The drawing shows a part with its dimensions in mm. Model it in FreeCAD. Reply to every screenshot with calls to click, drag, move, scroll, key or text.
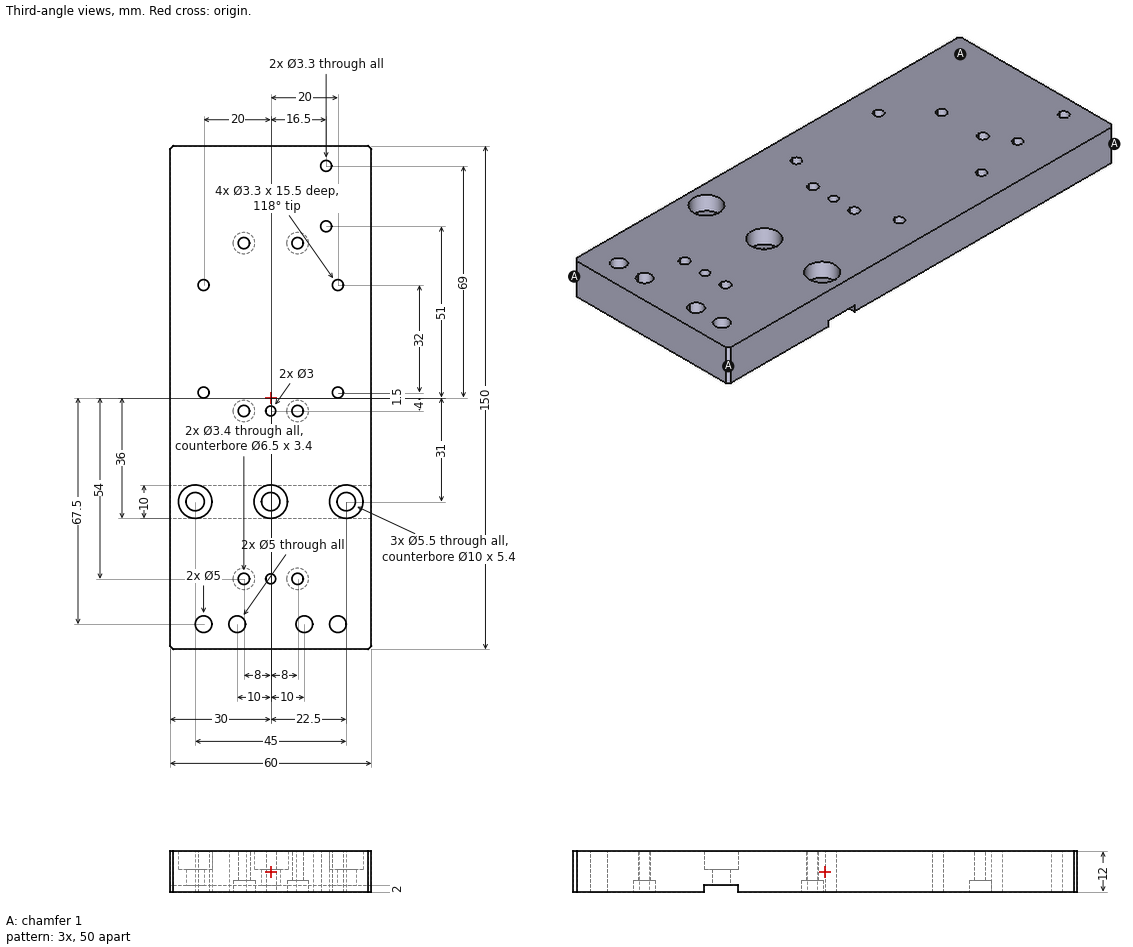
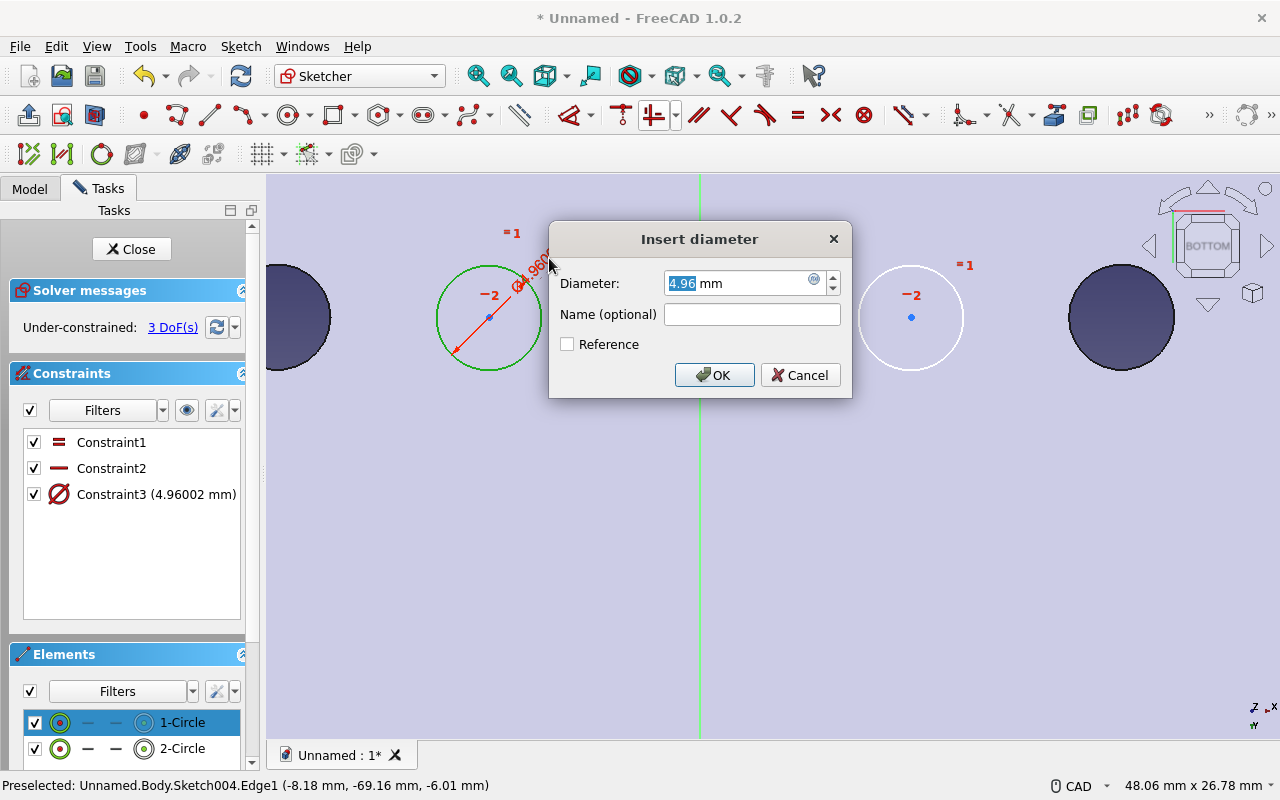
text(5)
key(Return)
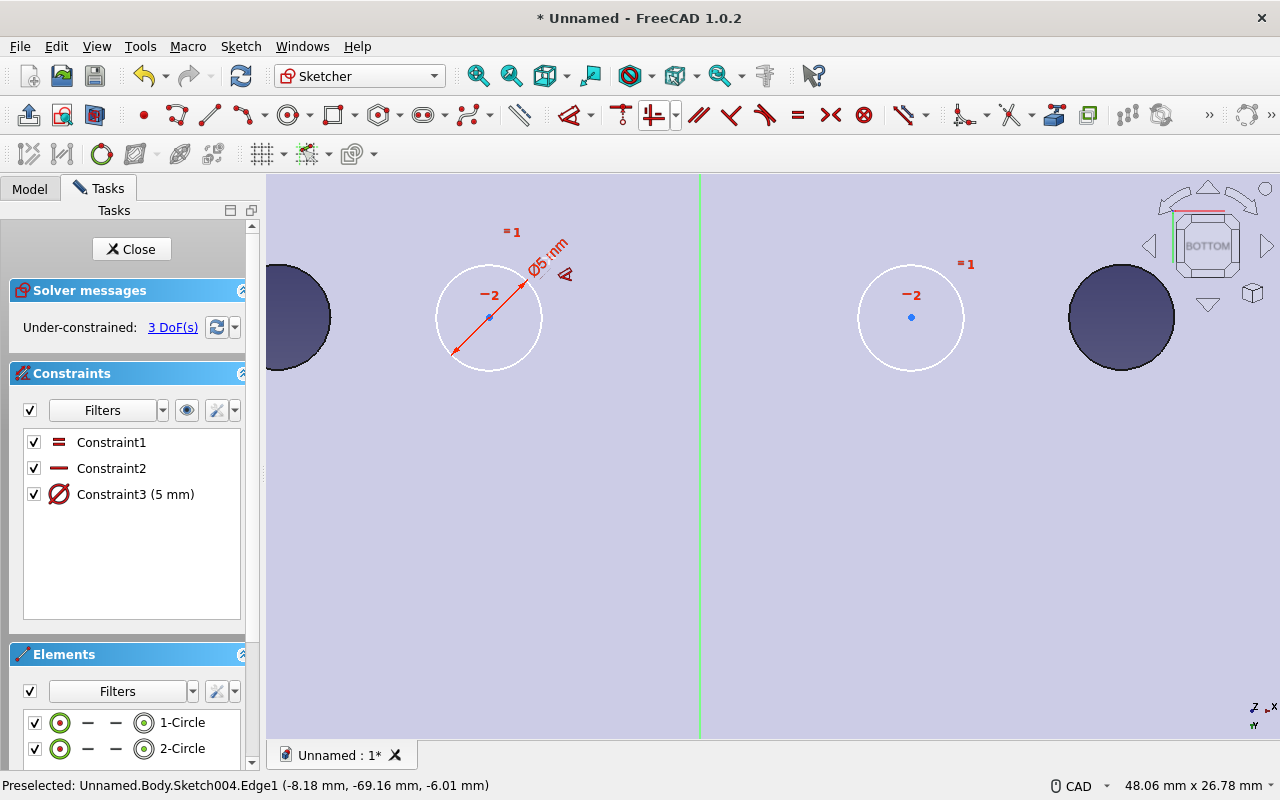
click(489, 318)
click(594, 284)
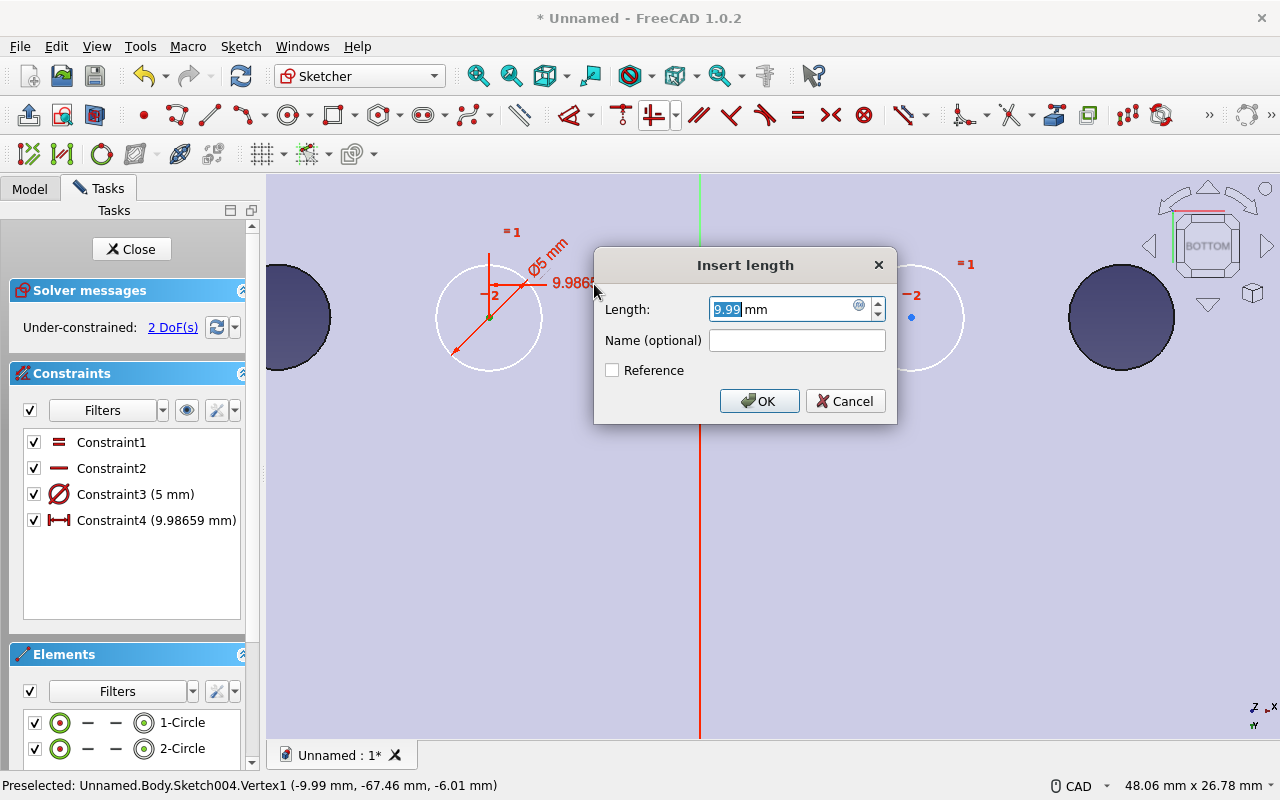
text(10)
key(Return)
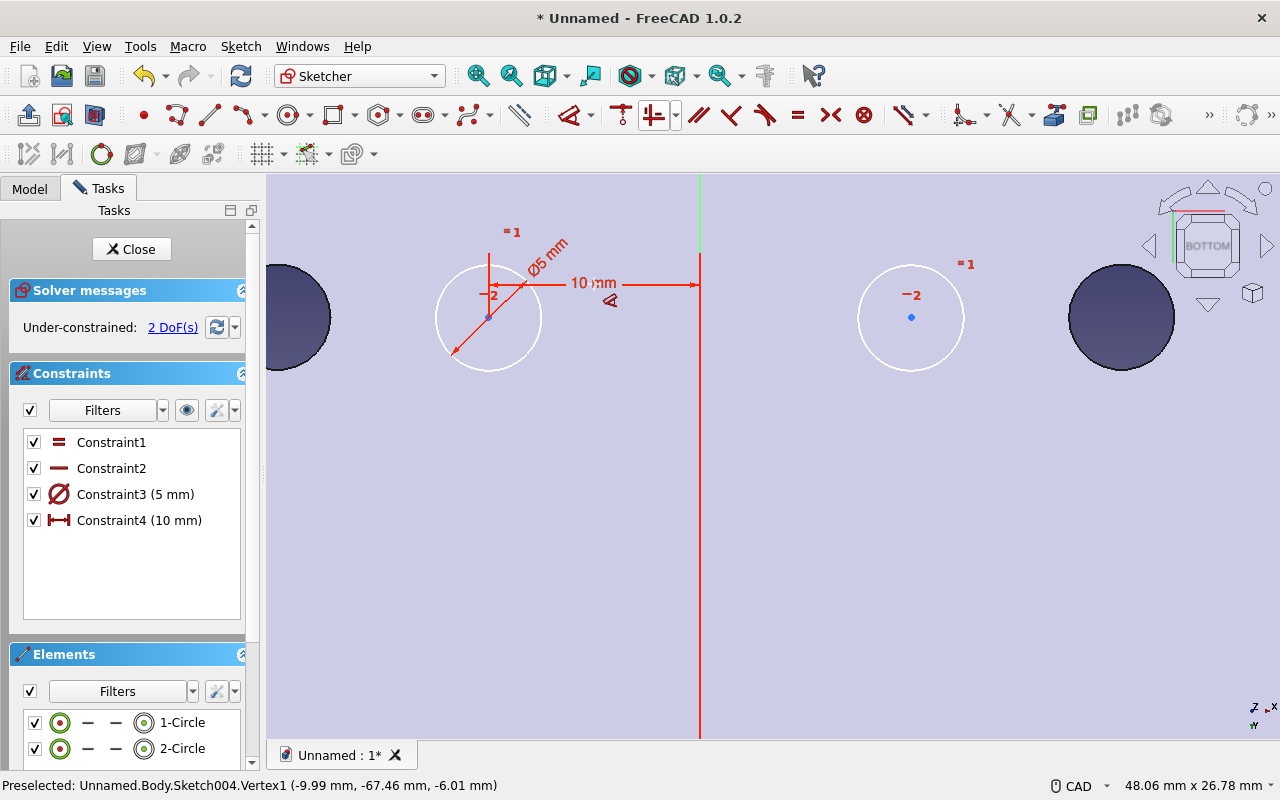
click(911, 318)
click(805, 284)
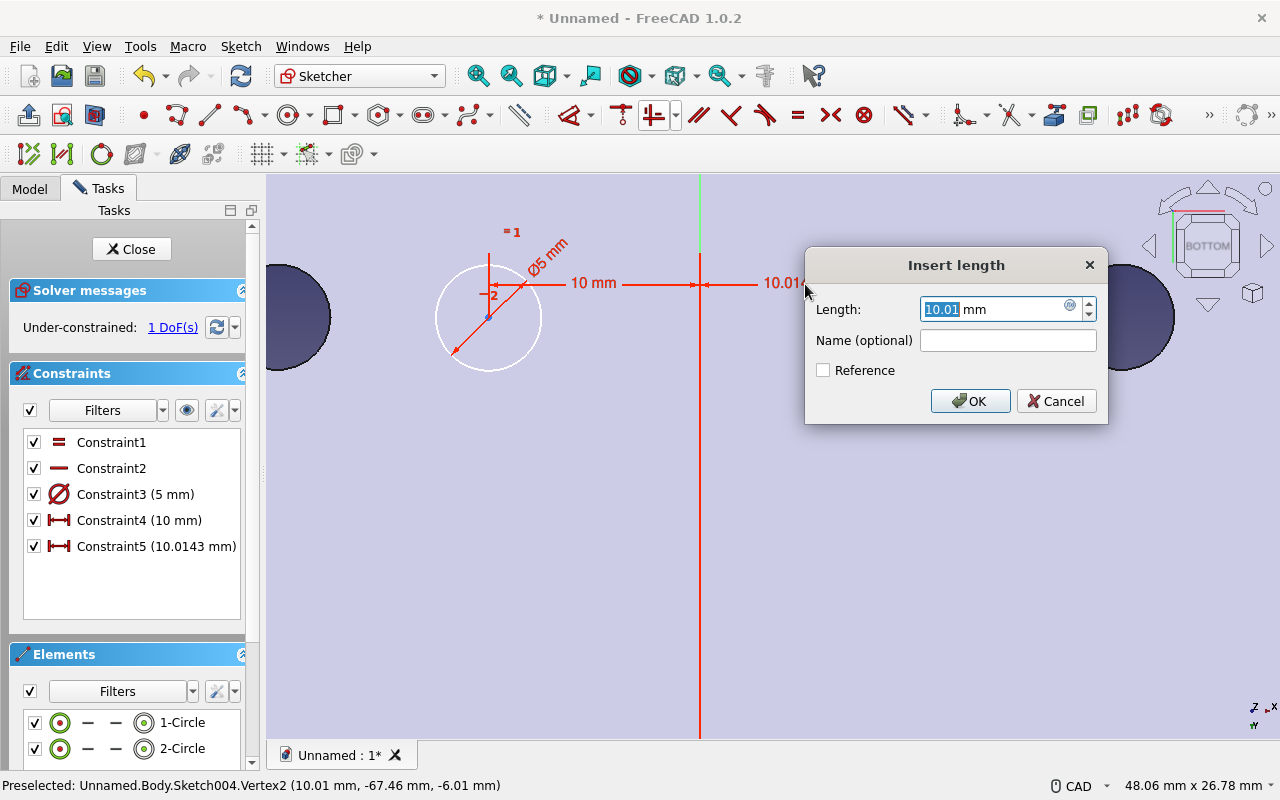
text(10)
key(Return)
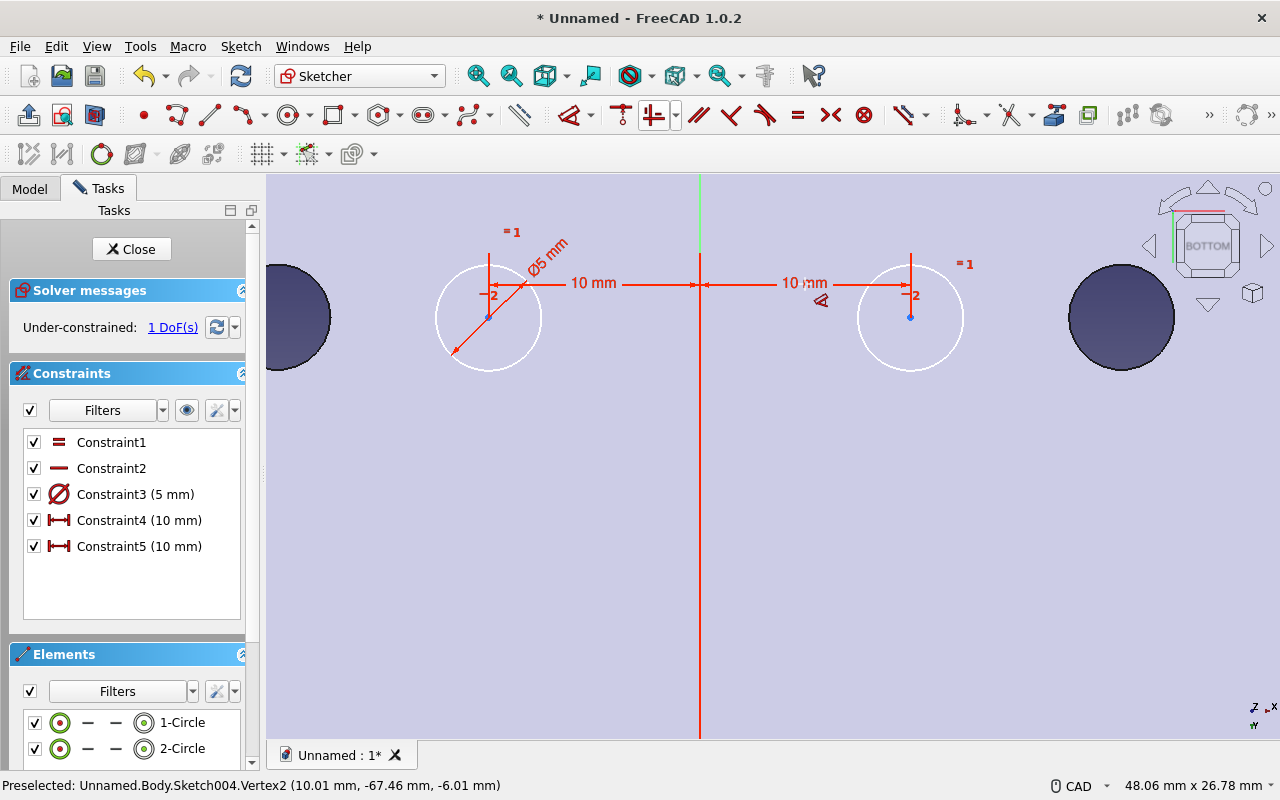
click(489, 318)
click(455, 514)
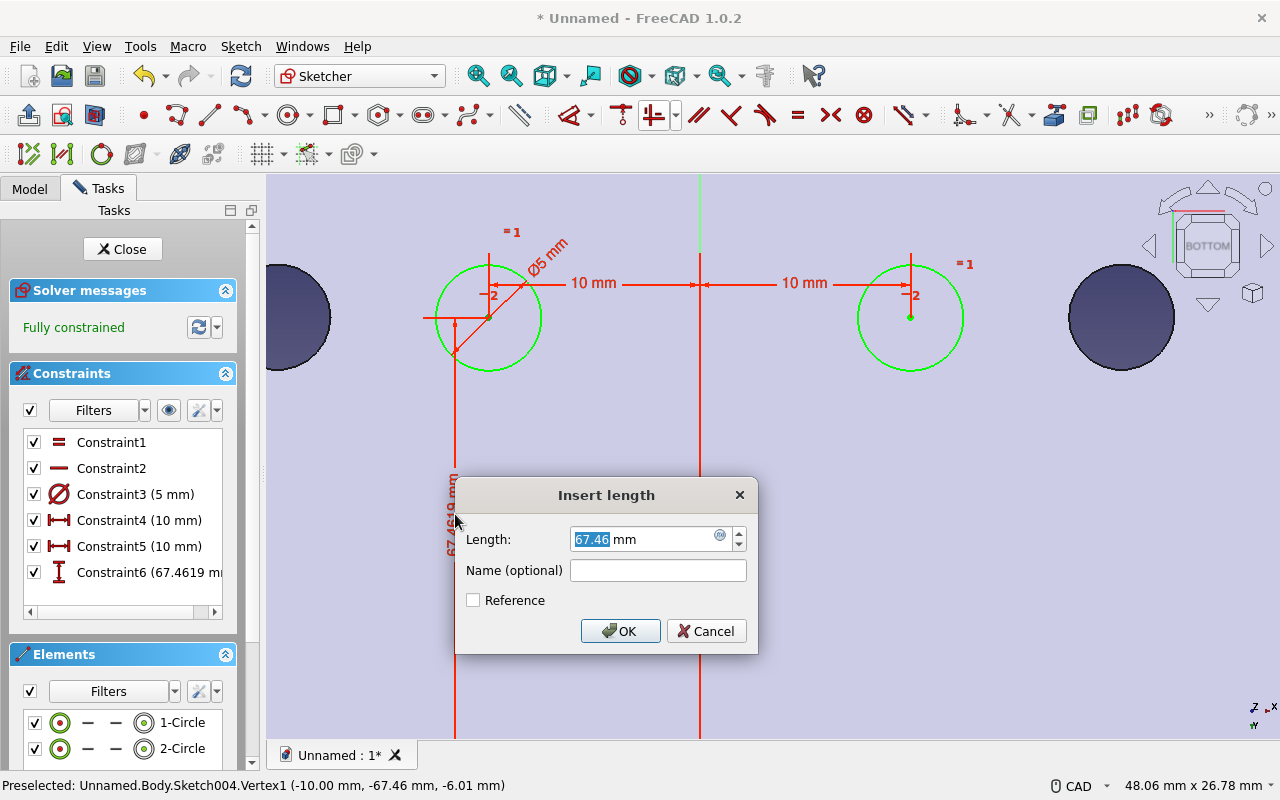
text(67.5)
key(Return)
key(Escape)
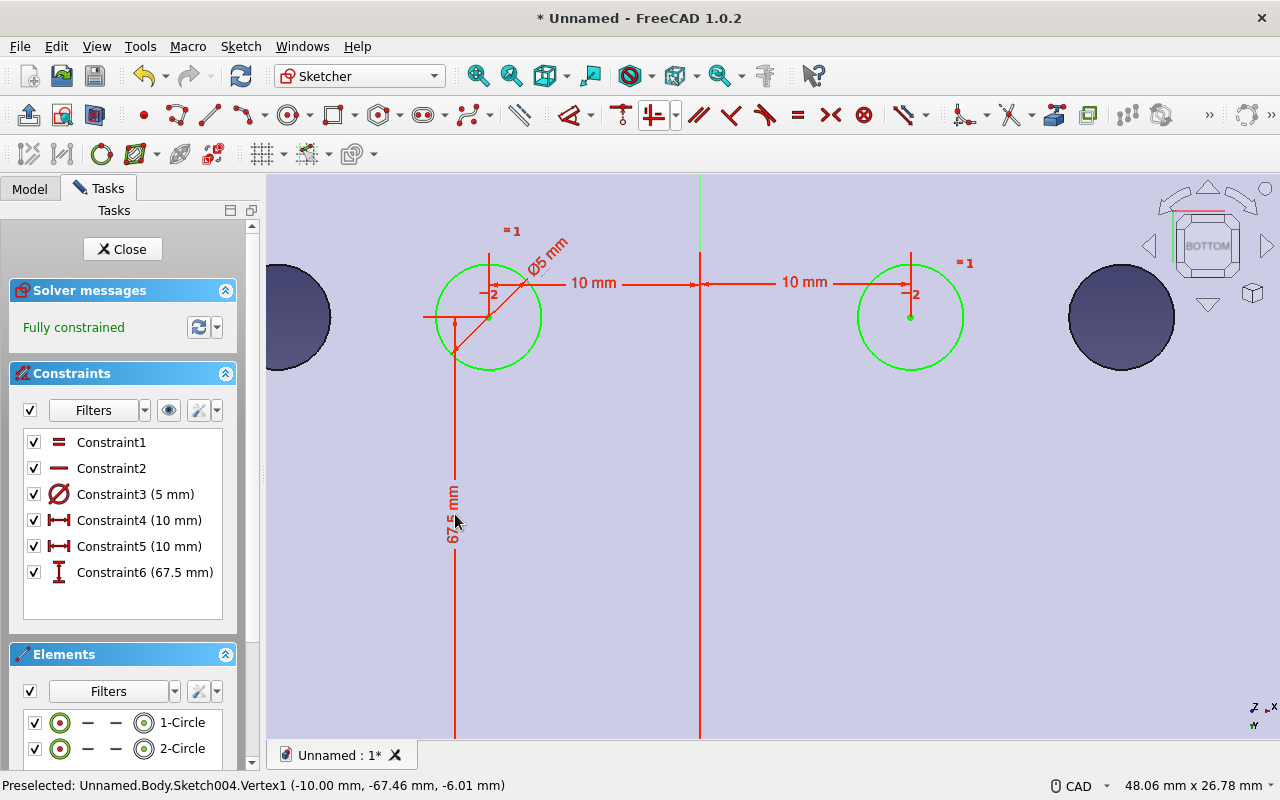
click(123, 249)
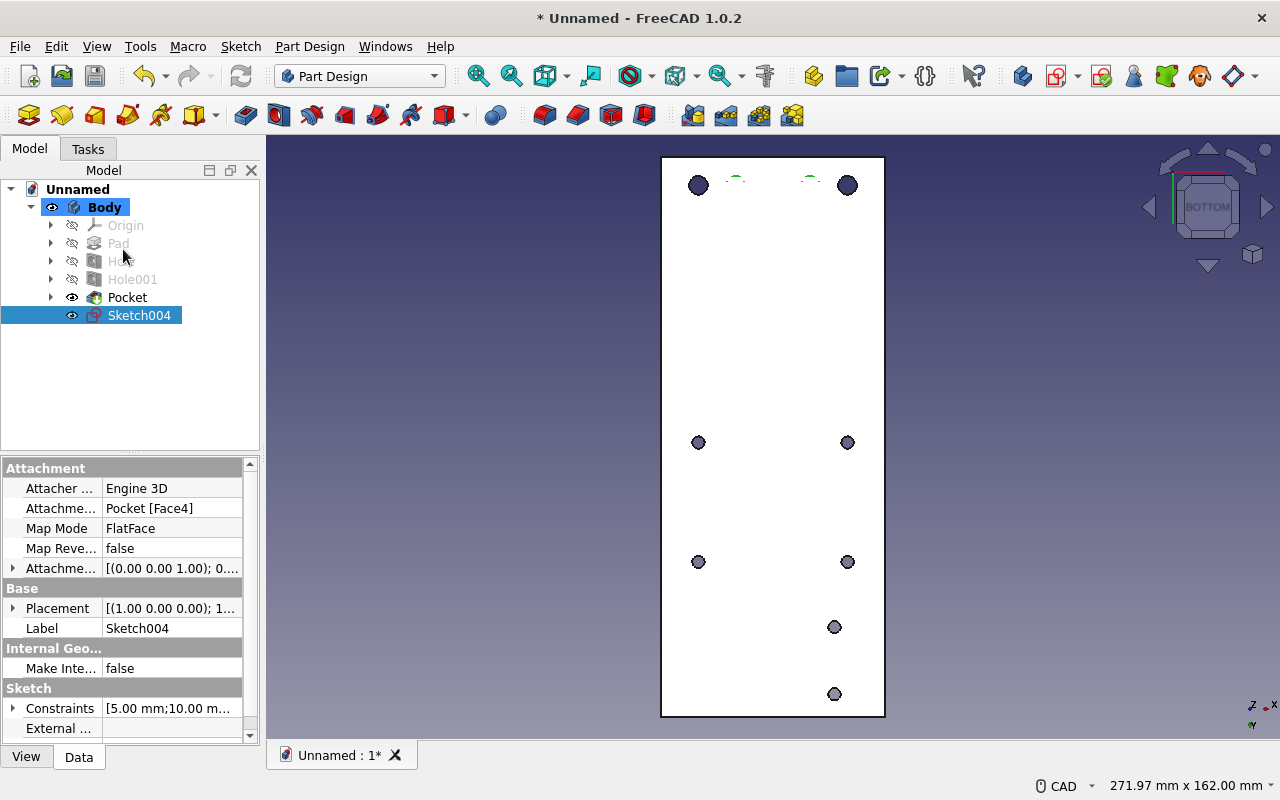
click(279, 116)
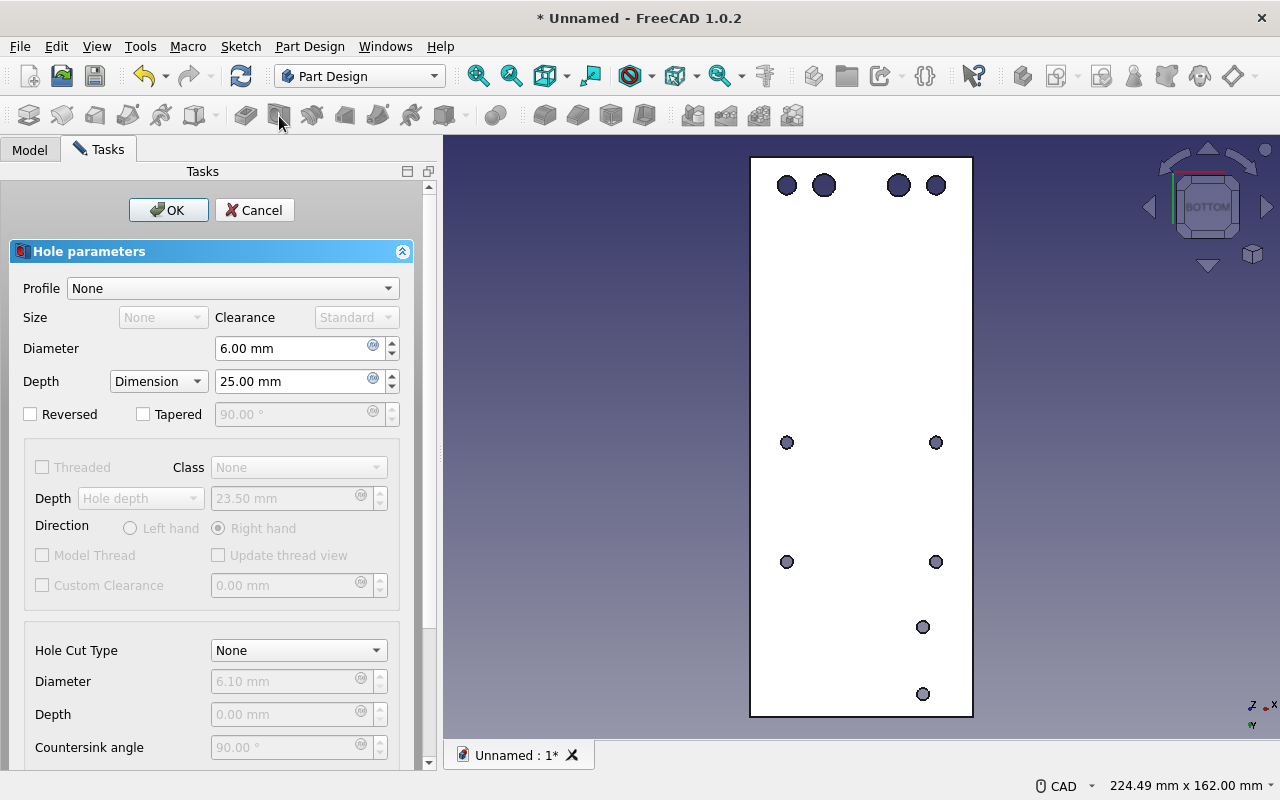
triple_click(300, 348)